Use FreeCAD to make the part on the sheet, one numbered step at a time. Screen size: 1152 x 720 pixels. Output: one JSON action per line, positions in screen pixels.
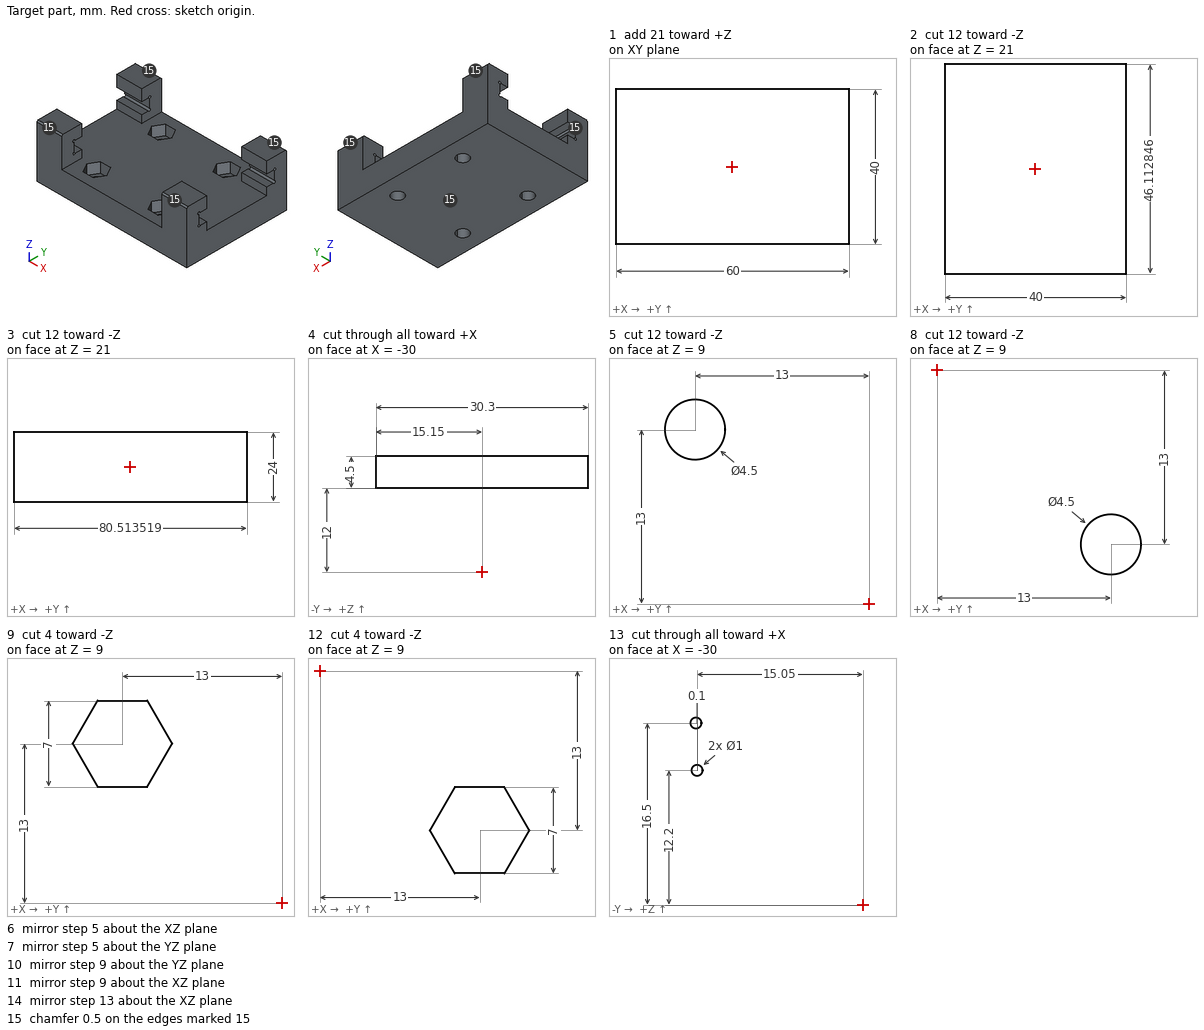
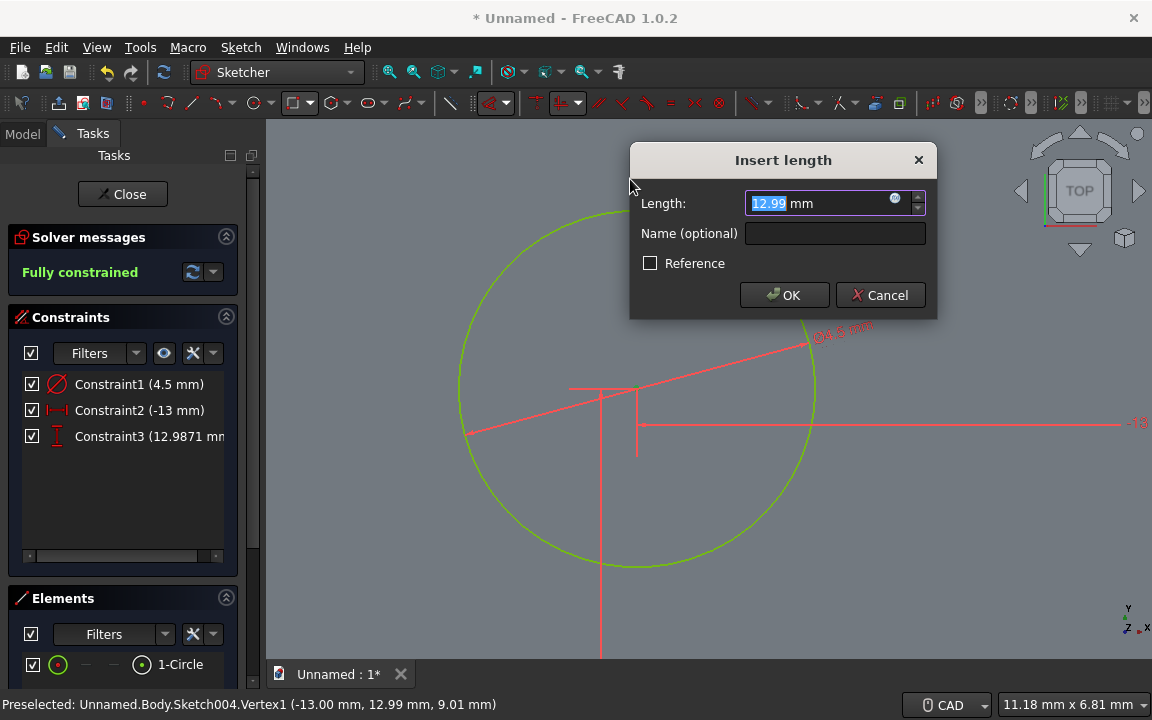
{"action": "type", "text": "13"}
{"action": "key", "text": "Return"}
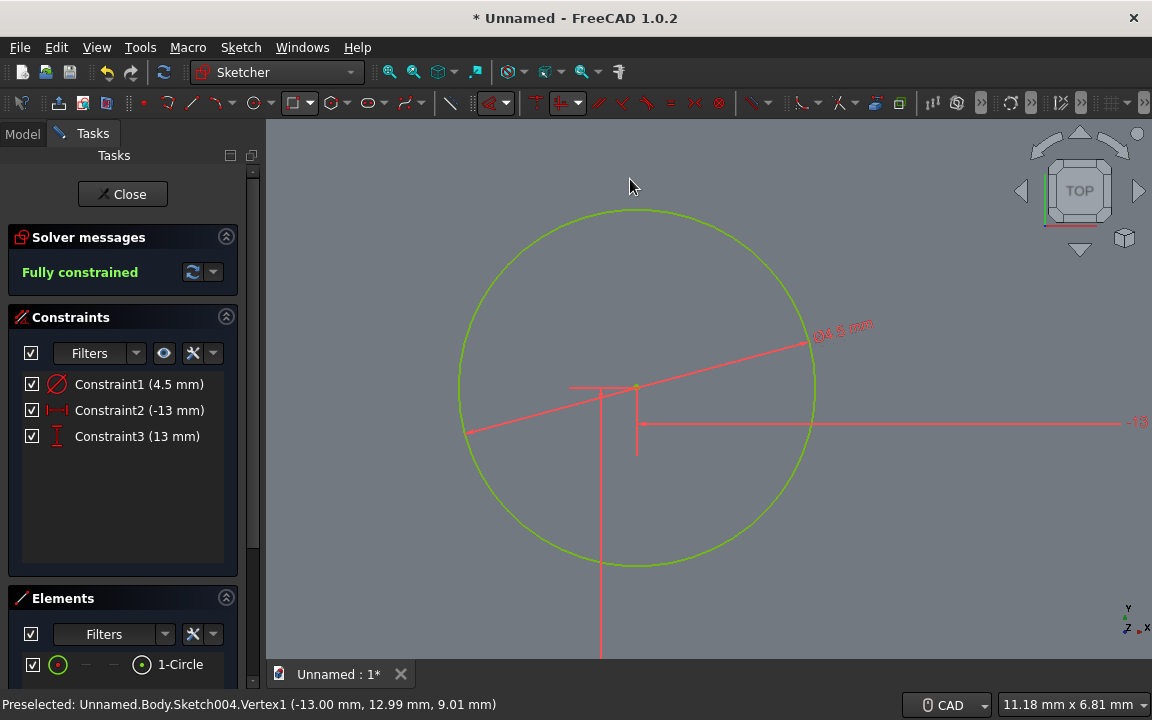
{"action": "left_click", "coordinate": [123, 194]}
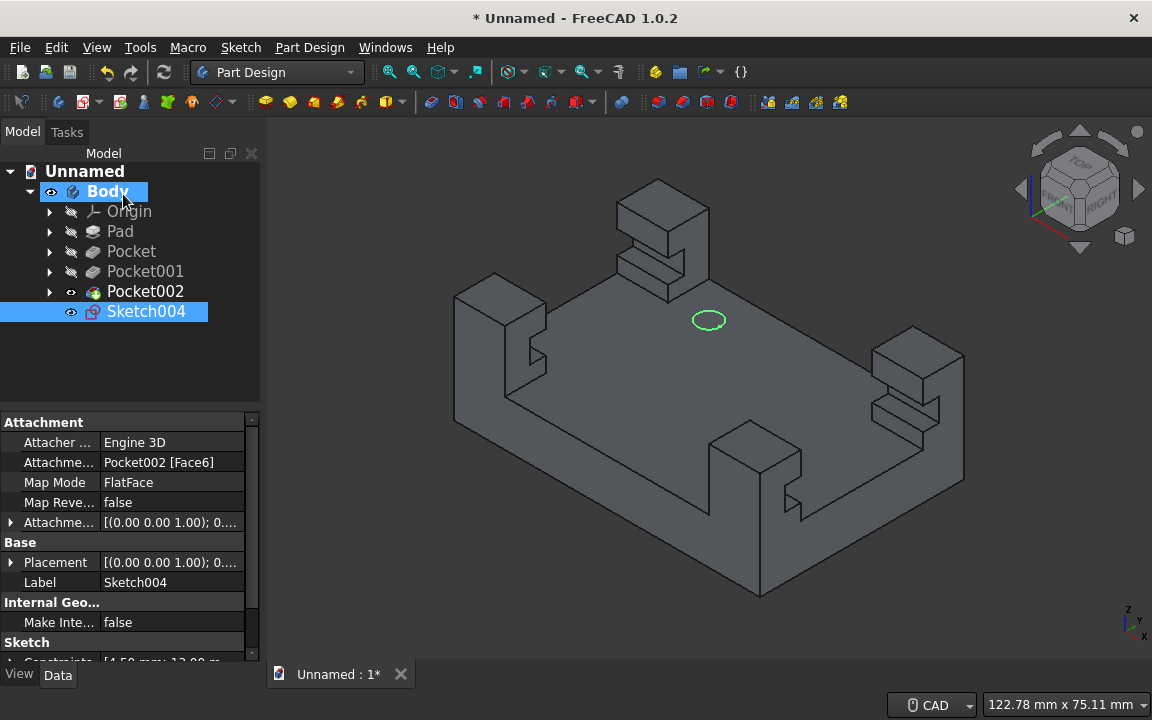
{"action": "left_click", "coordinate": [432, 102]}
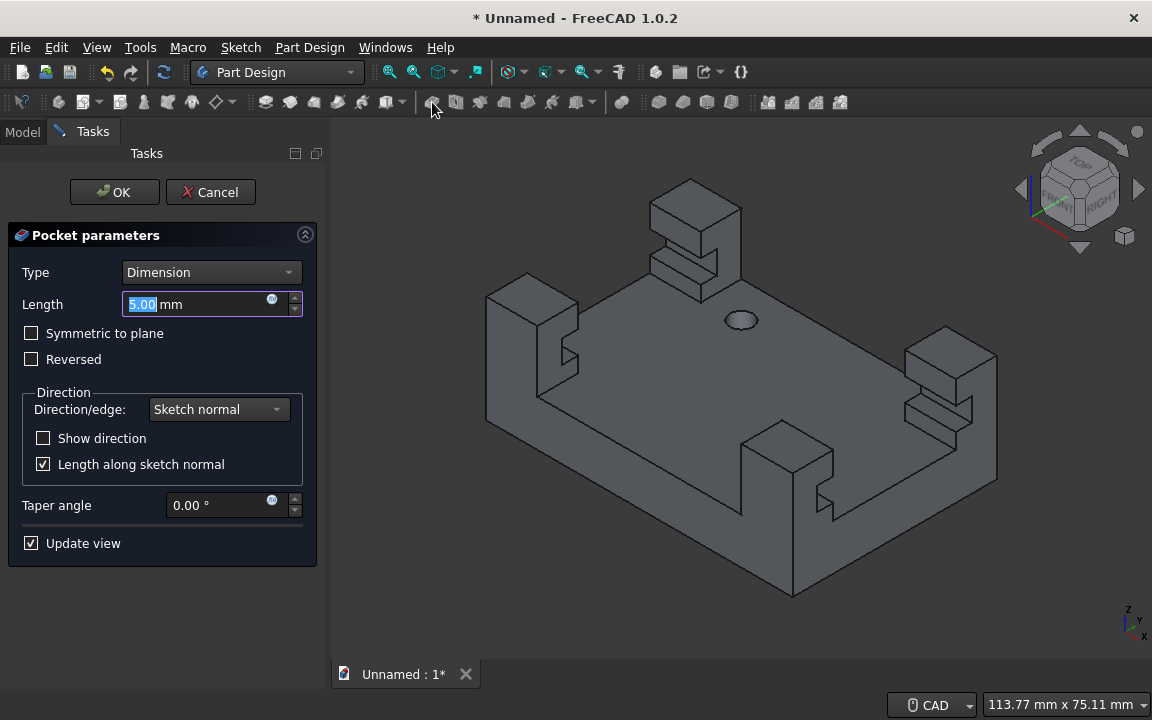
{"action": "type", "text": "12"}
{"action": "key", "text": "Tab"}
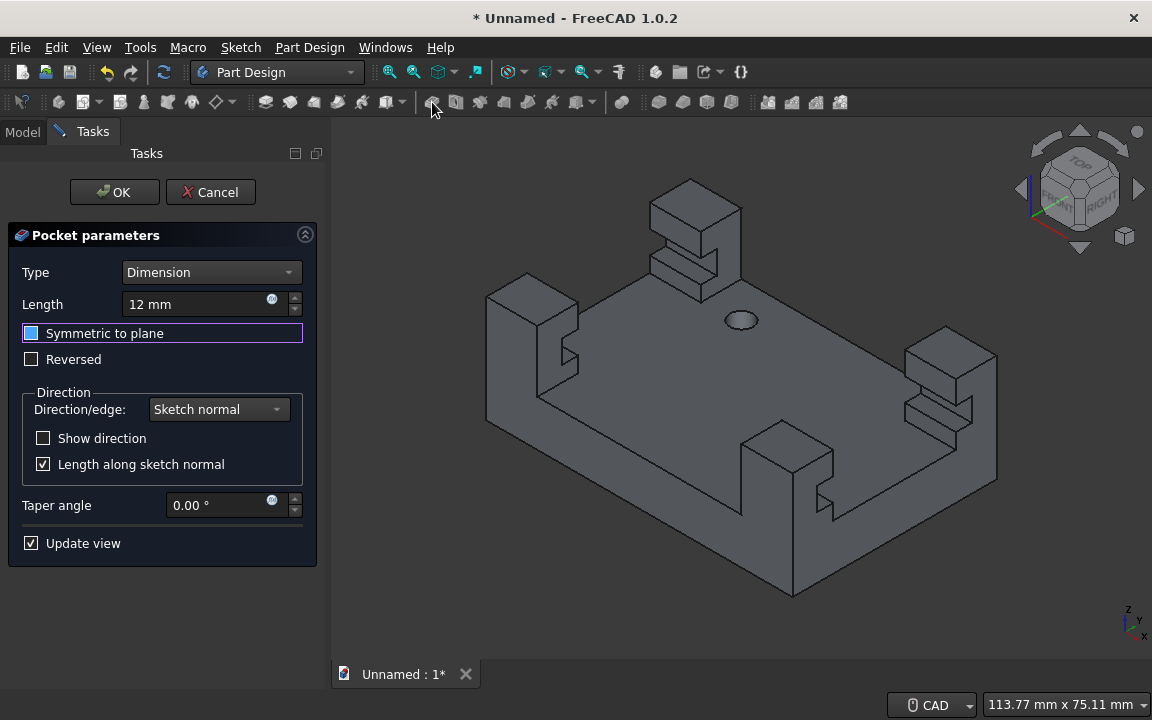
{"action": "left_click", "coordinate": [115, 192]}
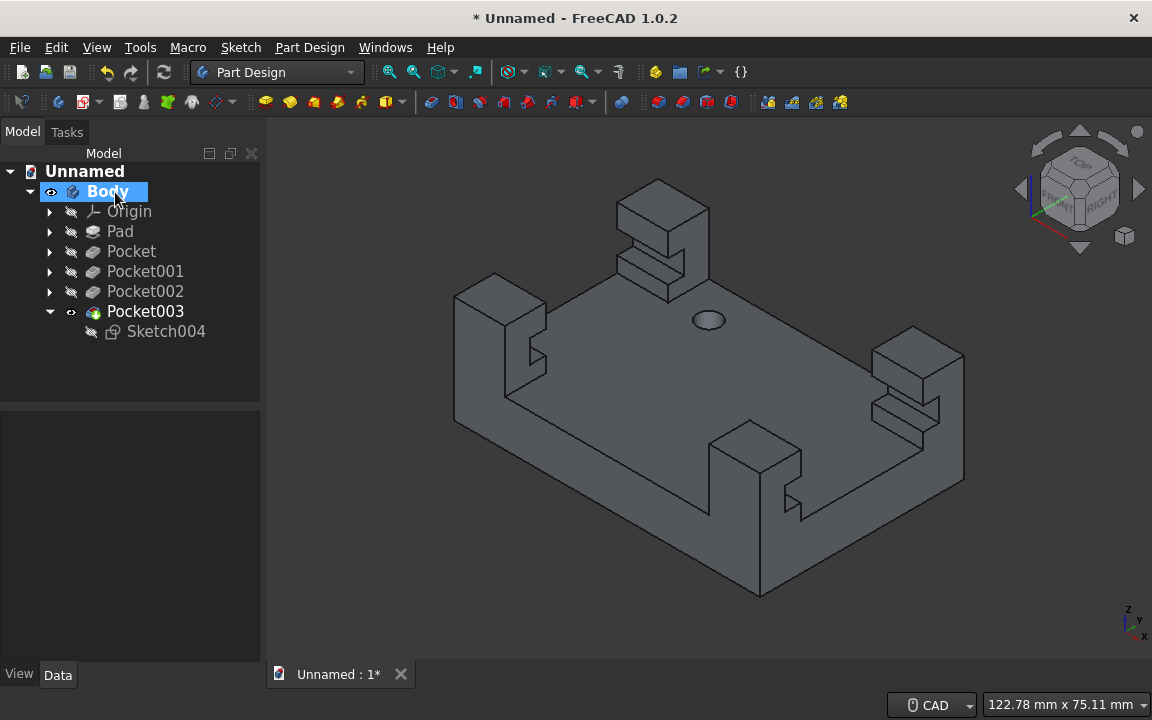
{"action": "left_click", "coordinate": [116, 312]}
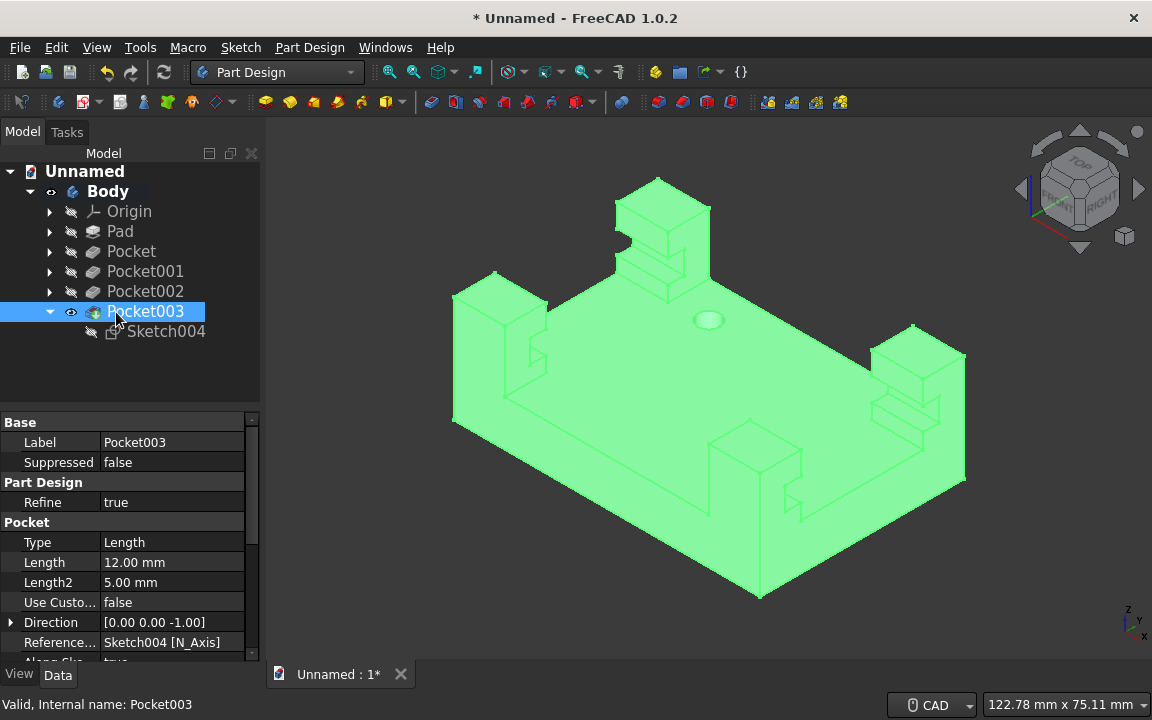
{"action": "left_click", "coordinate": [768, 102]}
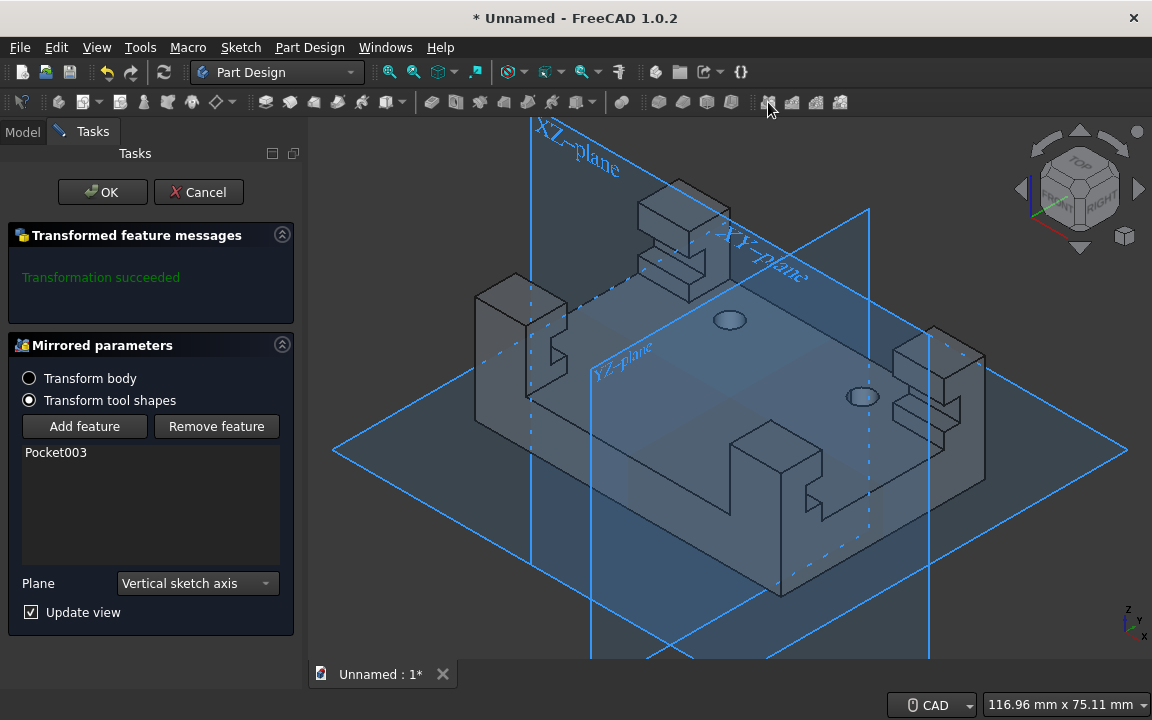
{"action": "left_click", "coordinate": [198, 584]}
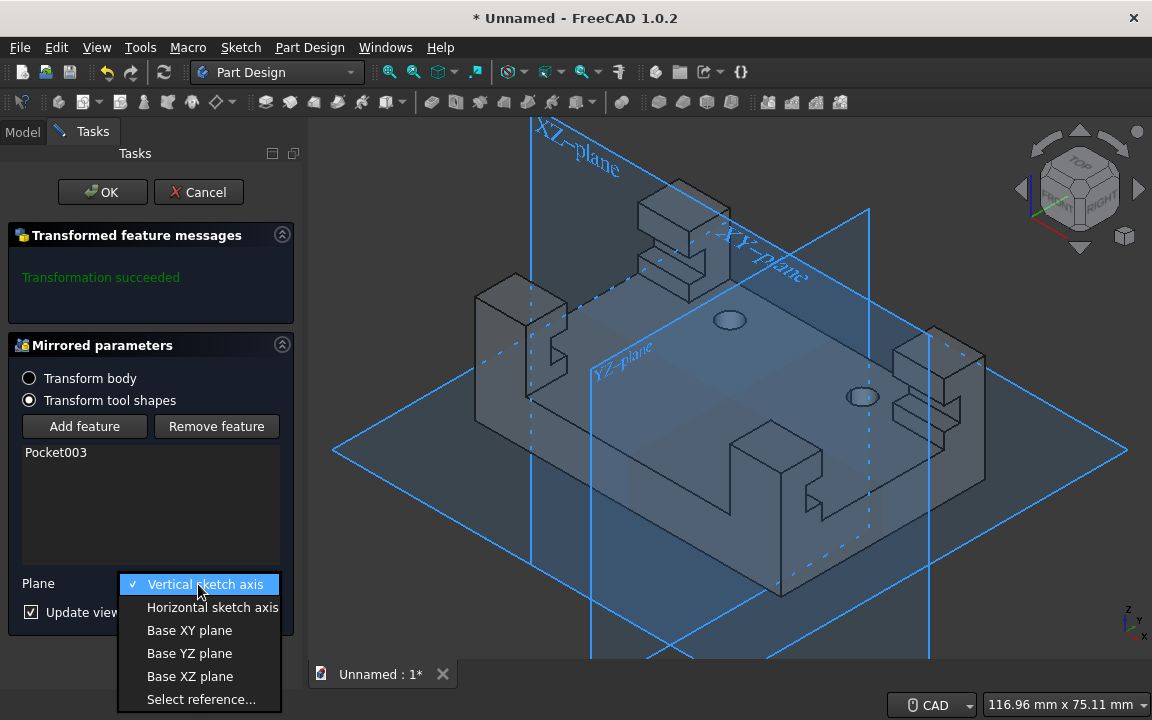
{"action": "left_click", "coordinate": [198, 676]}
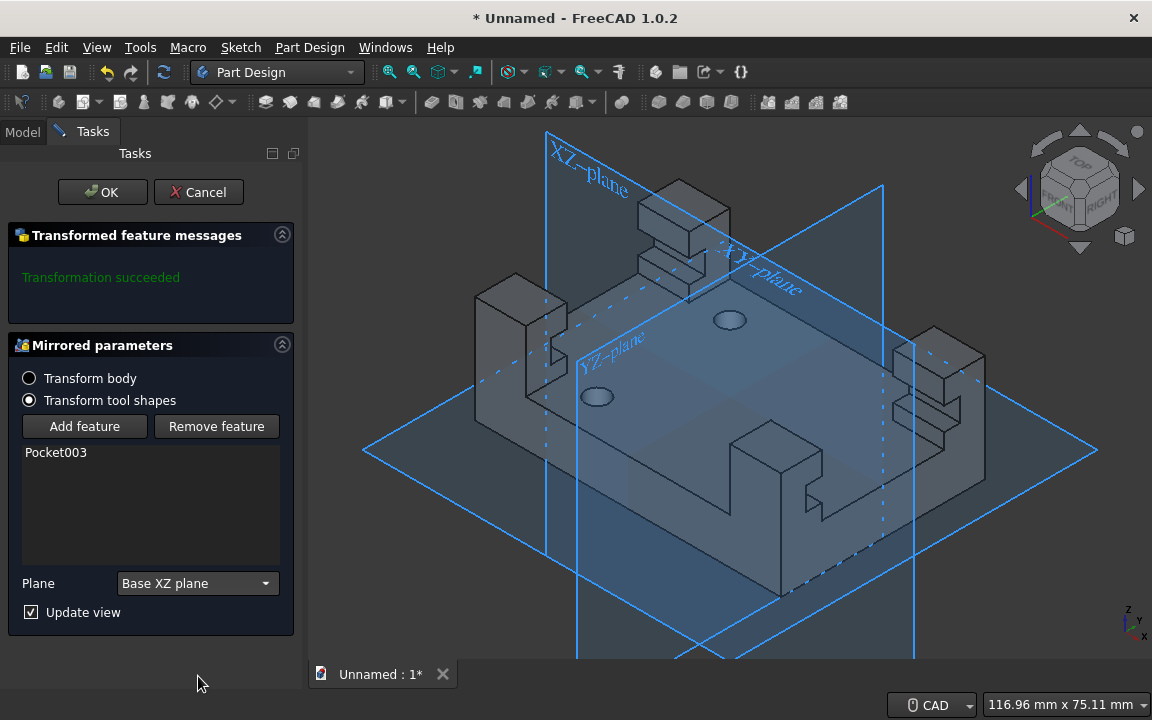
{"action": "left_click", "coordinate": [103, 192]}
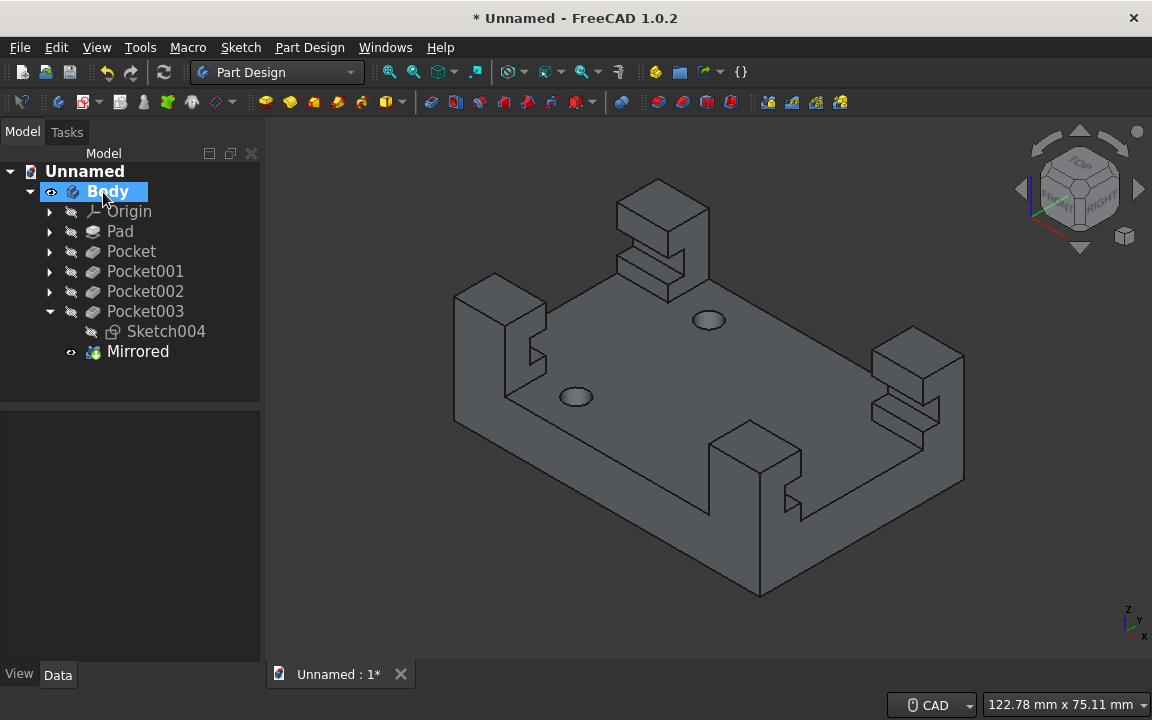
{"action": "left_click", "coordinate": [116, 312]}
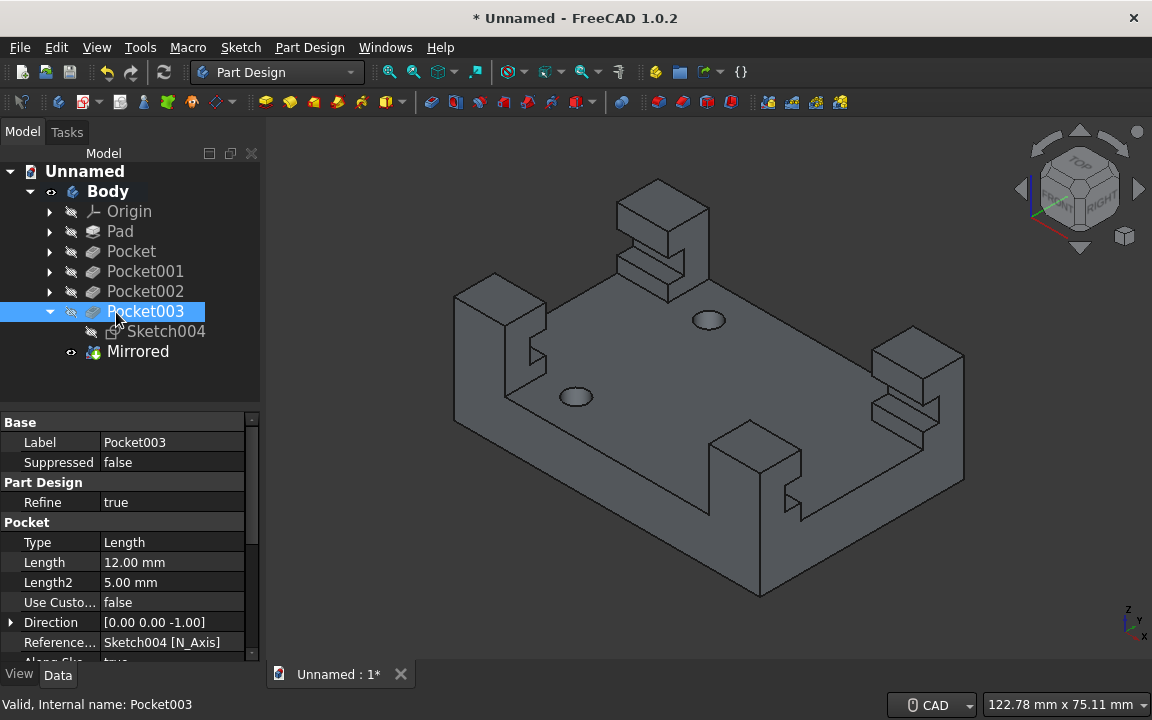
{"action": "left_click", "coordinate": [768, 102]}